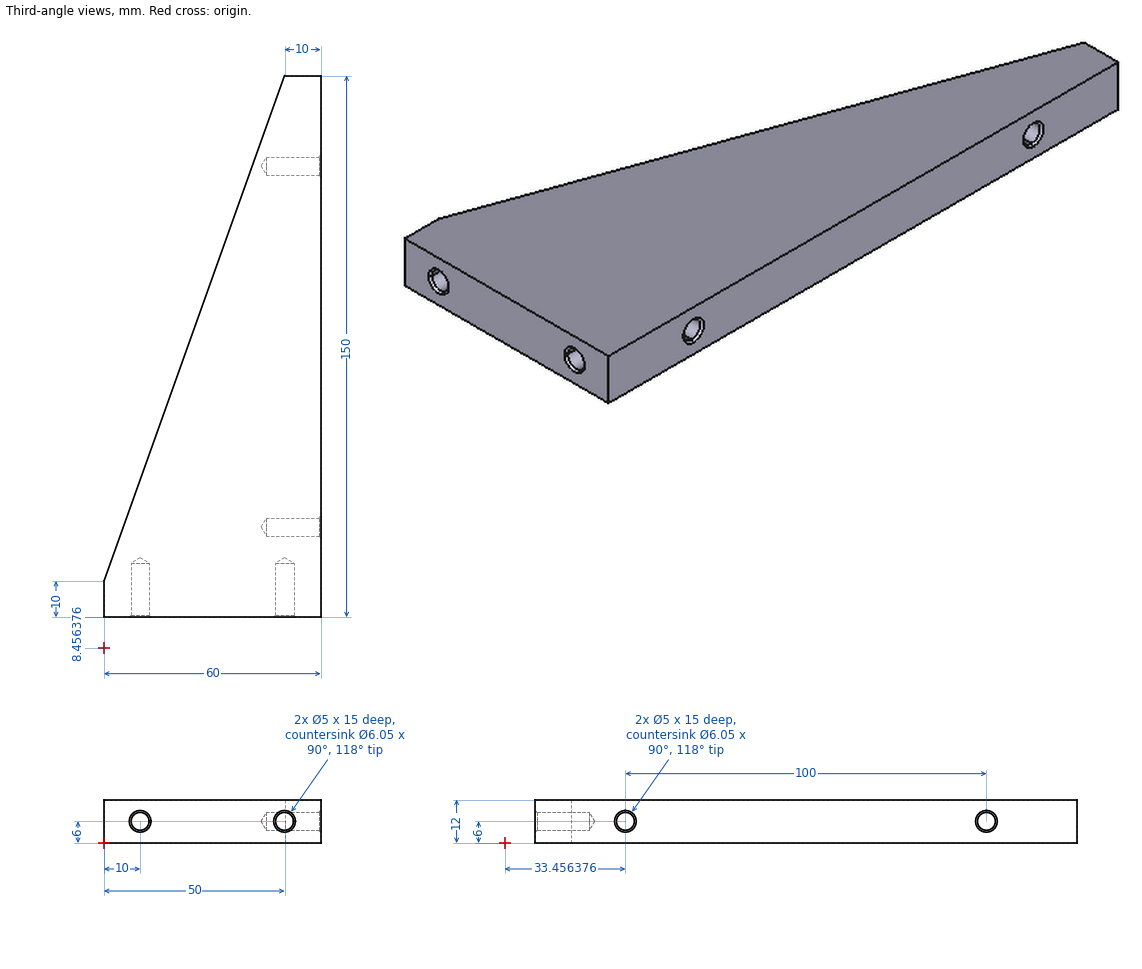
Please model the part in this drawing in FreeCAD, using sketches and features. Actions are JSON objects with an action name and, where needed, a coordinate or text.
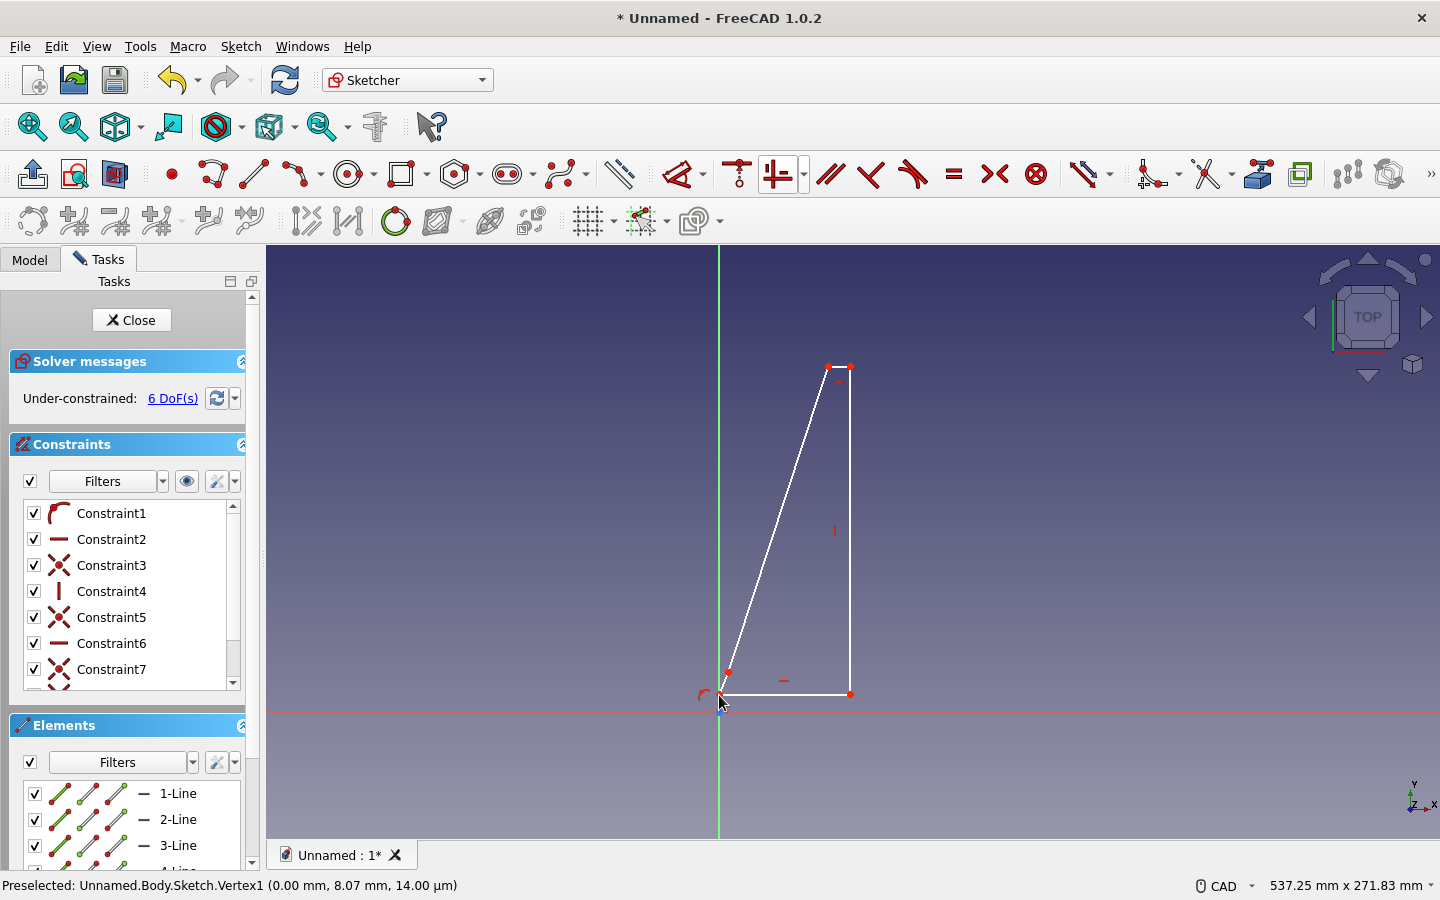
{"action": "scroll", "coordinate": [723, 686], "scroll_direction": "up", "scroll_amount": 3}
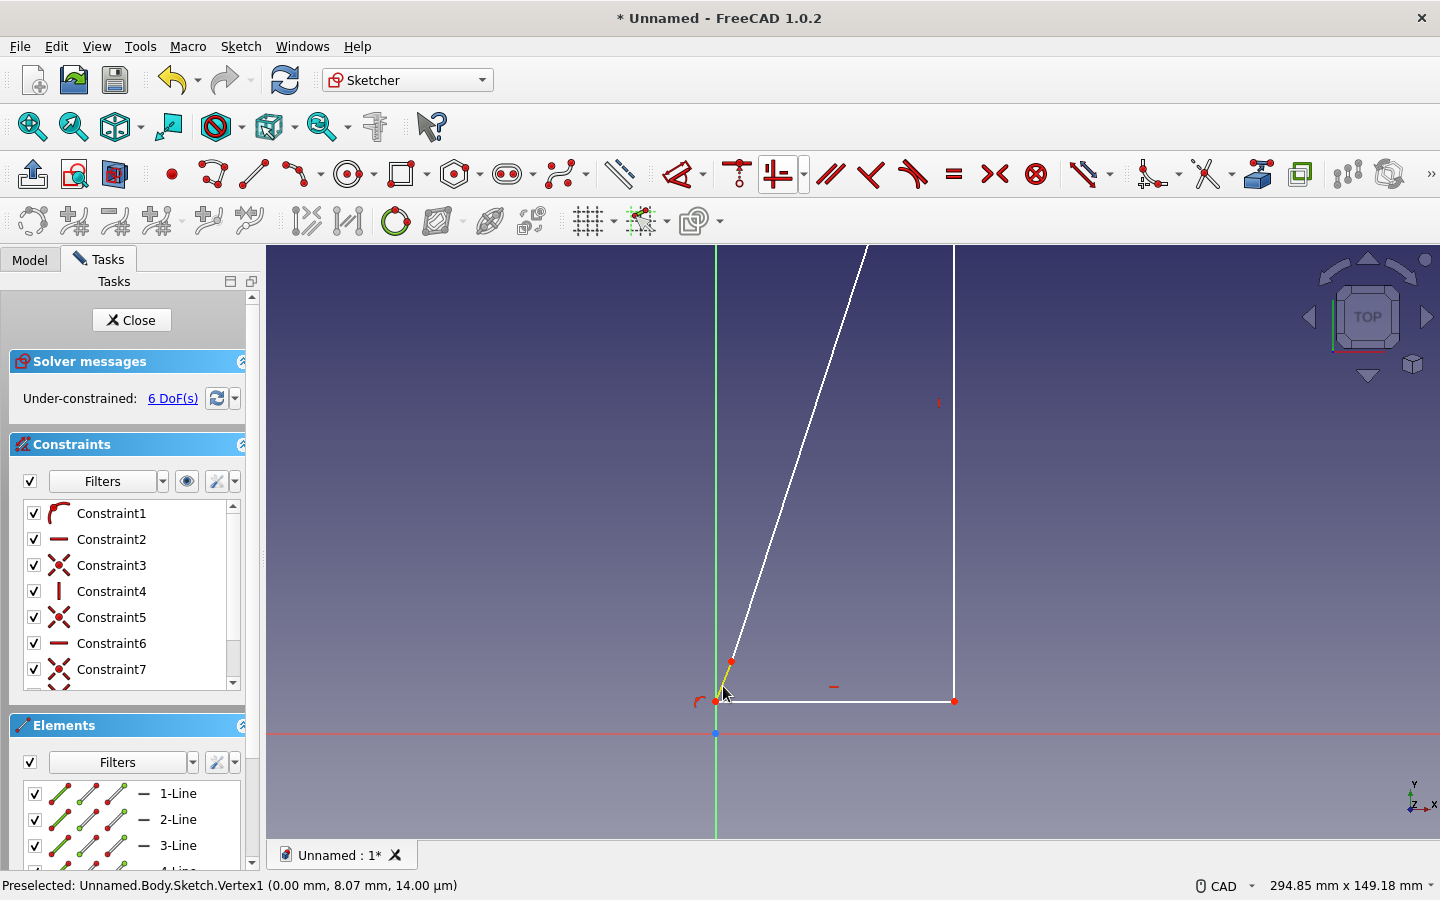
{"action": "left_click", "coordinate": [722, 686]}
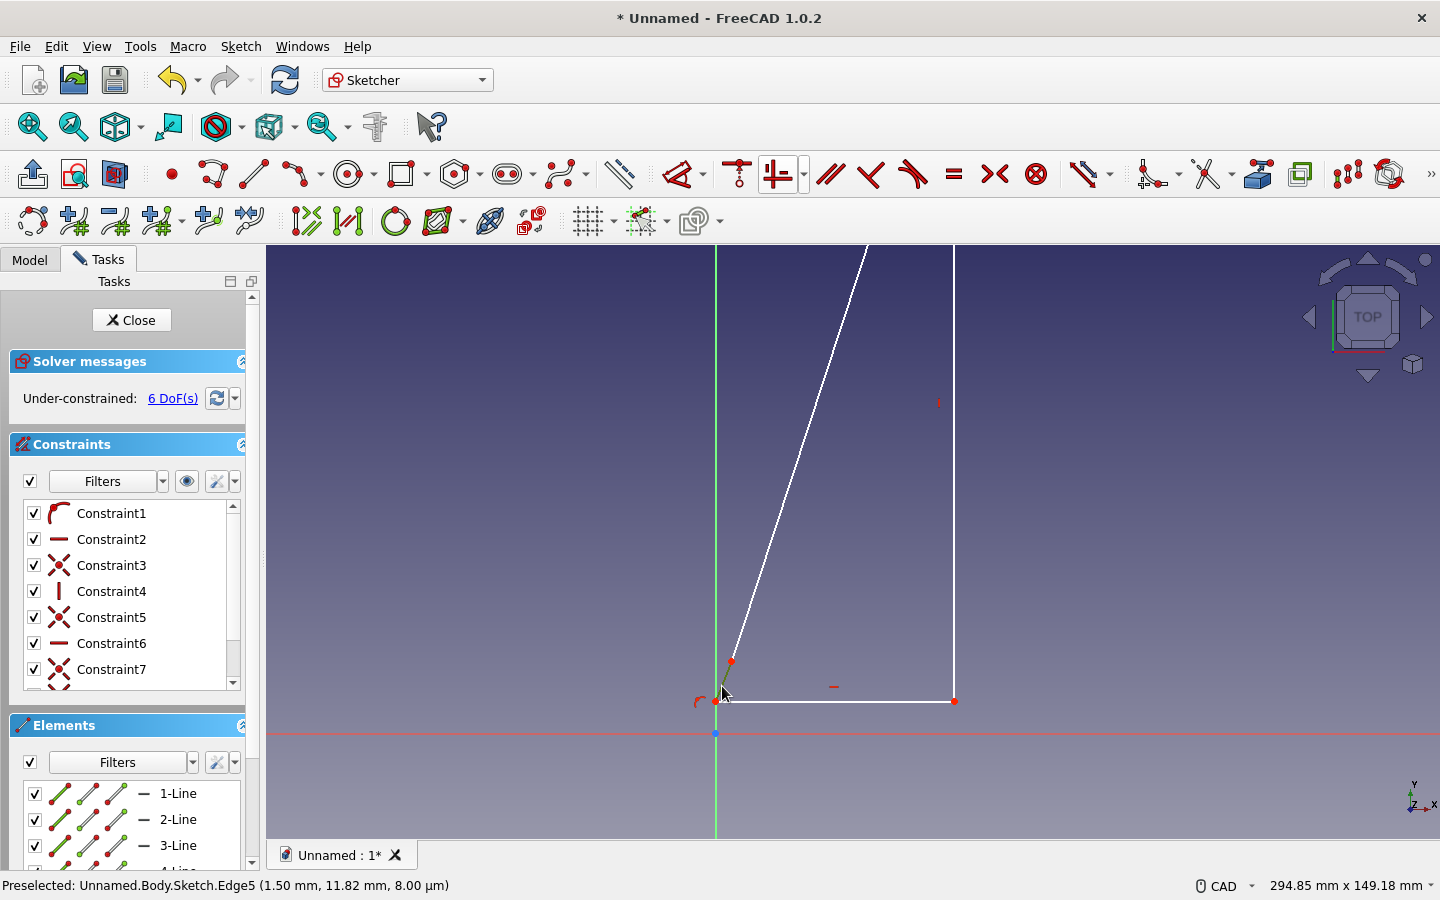
{"action": "key", "text": "v"}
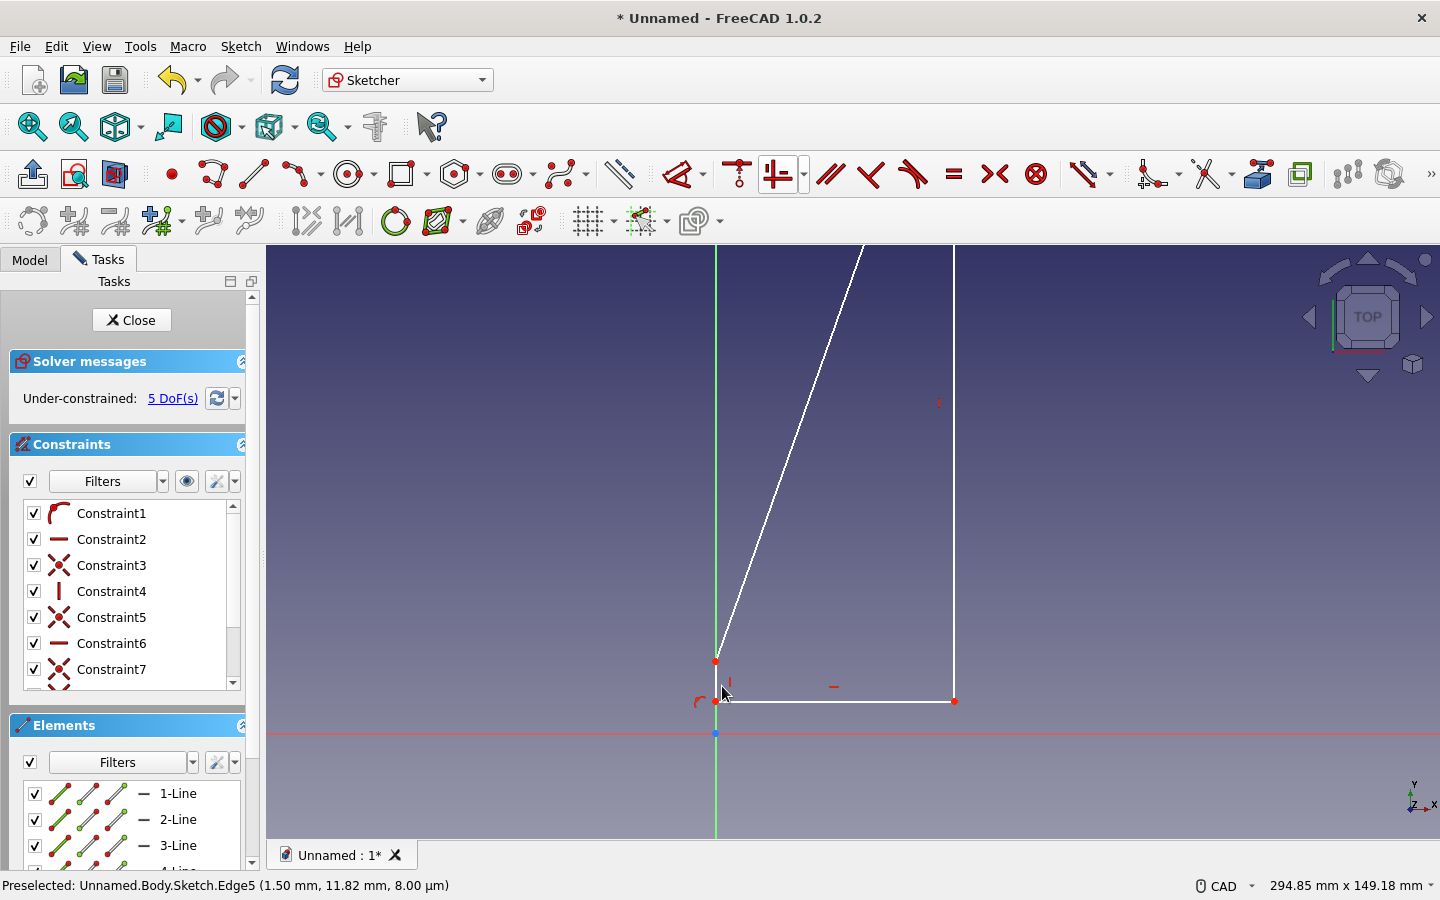
{"action": "left_click", "coordinate": [676, 174]}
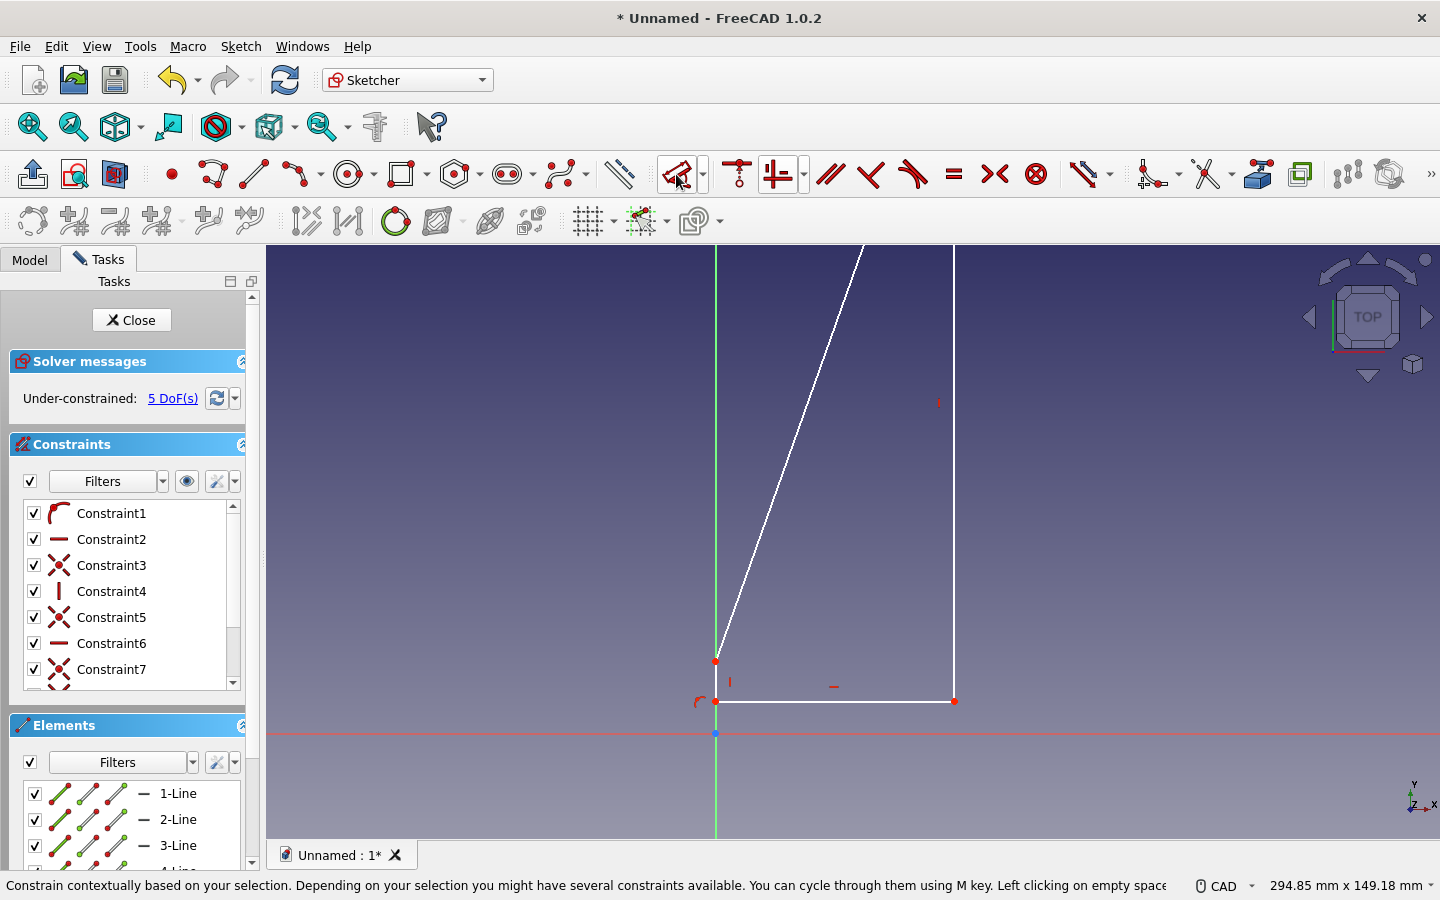
{"action": "left_click", "coordinate": [787, 702]}
{"action": "left_click", "coordinate": [835, 668]}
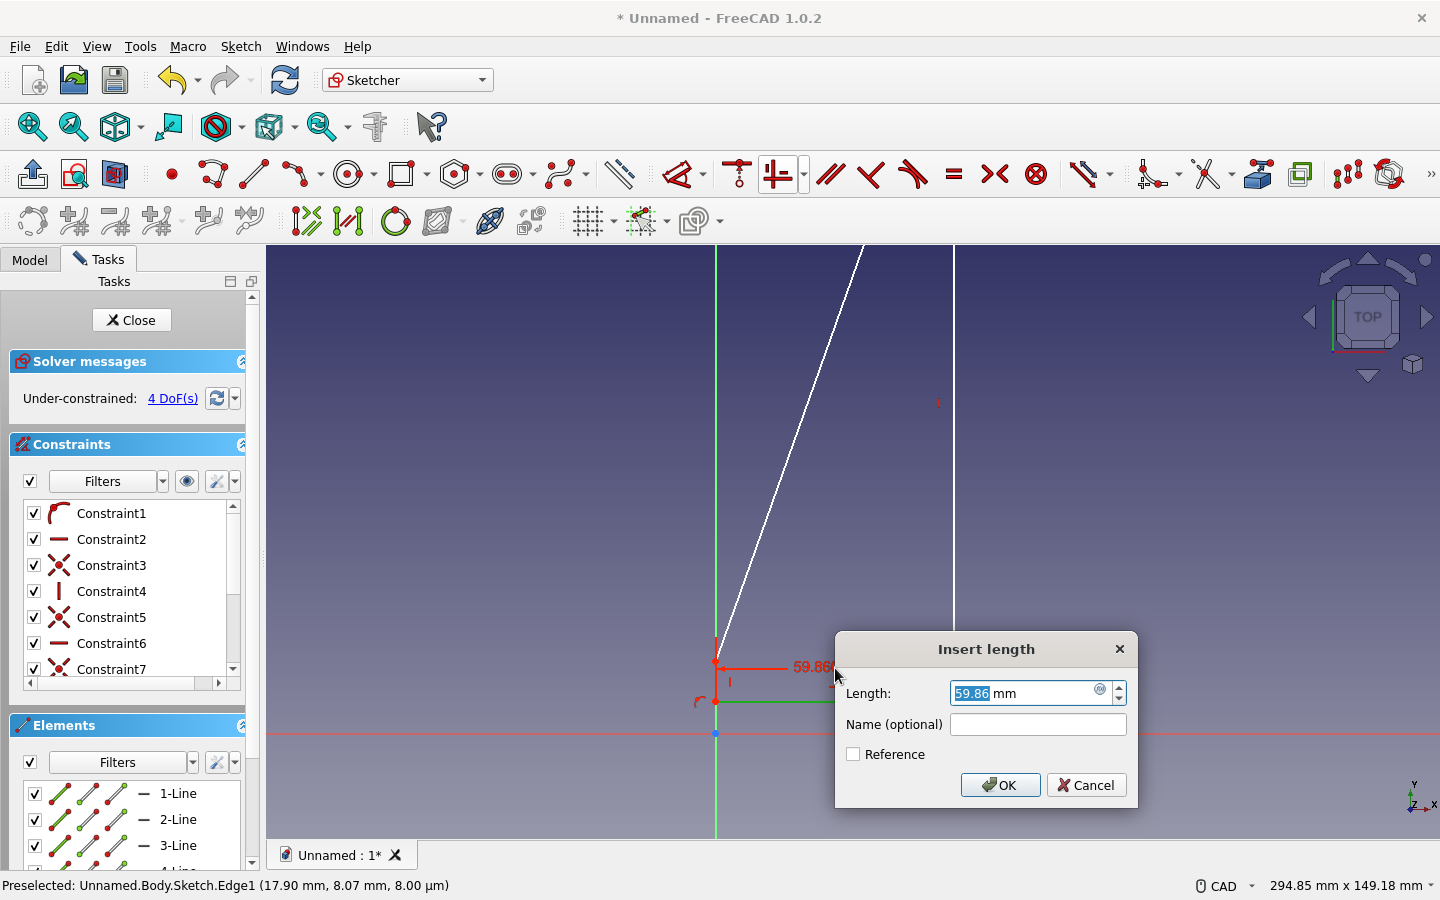
{"action": "type", "text": "60"}
{"action": "key", "text": "Return"}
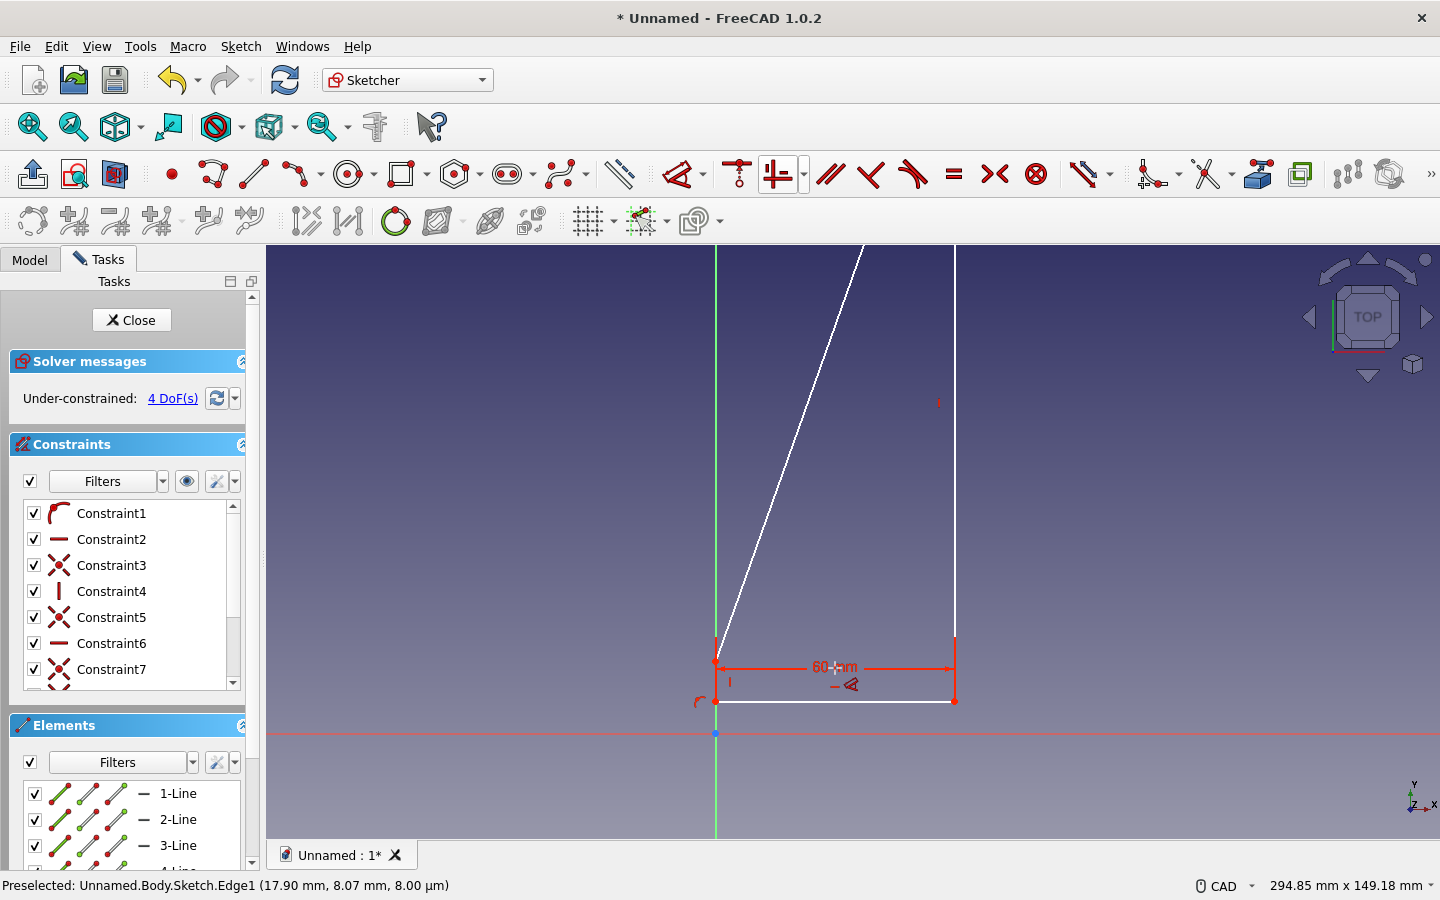
{"action": "scroll", "coordinate": [723, 692], "scroll_direction": "down", "scroll_amount": 3}